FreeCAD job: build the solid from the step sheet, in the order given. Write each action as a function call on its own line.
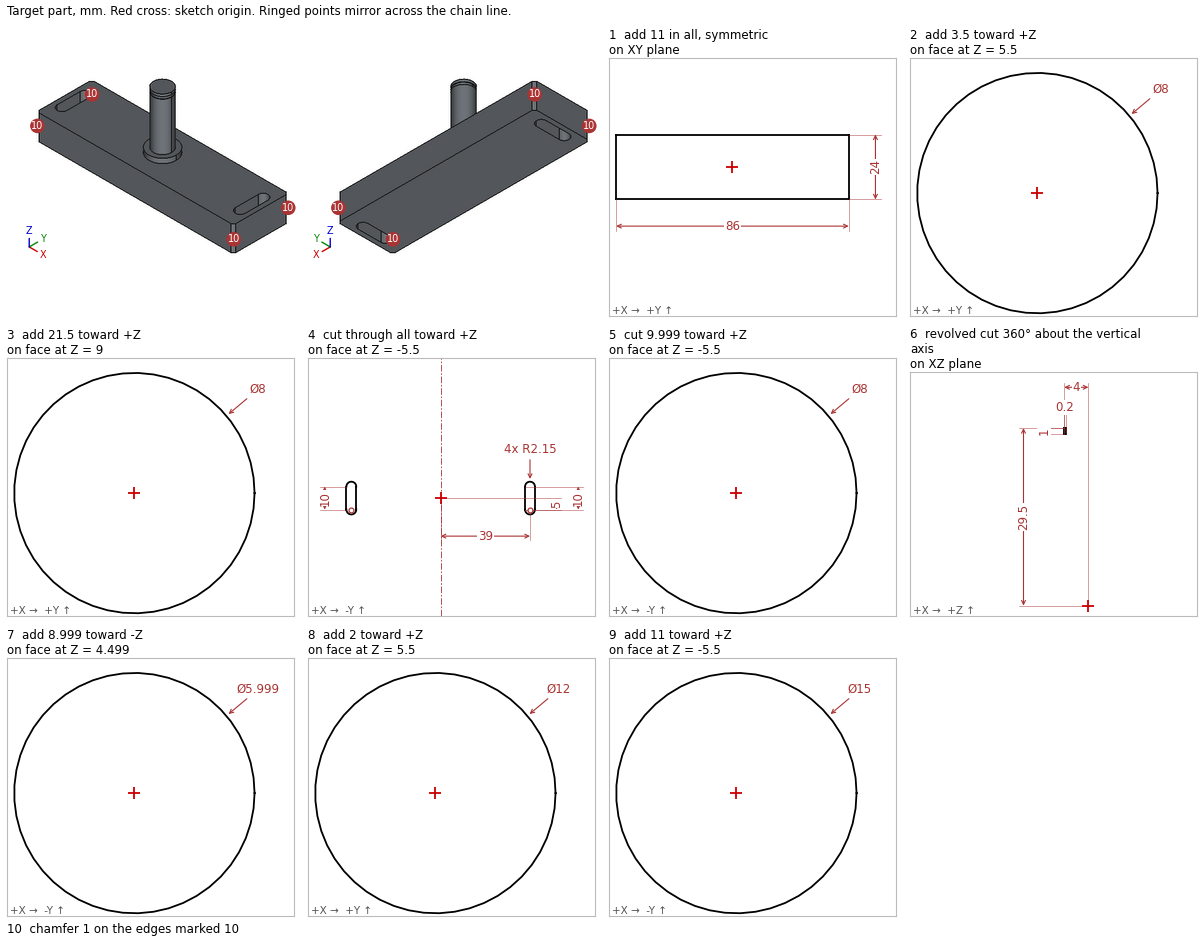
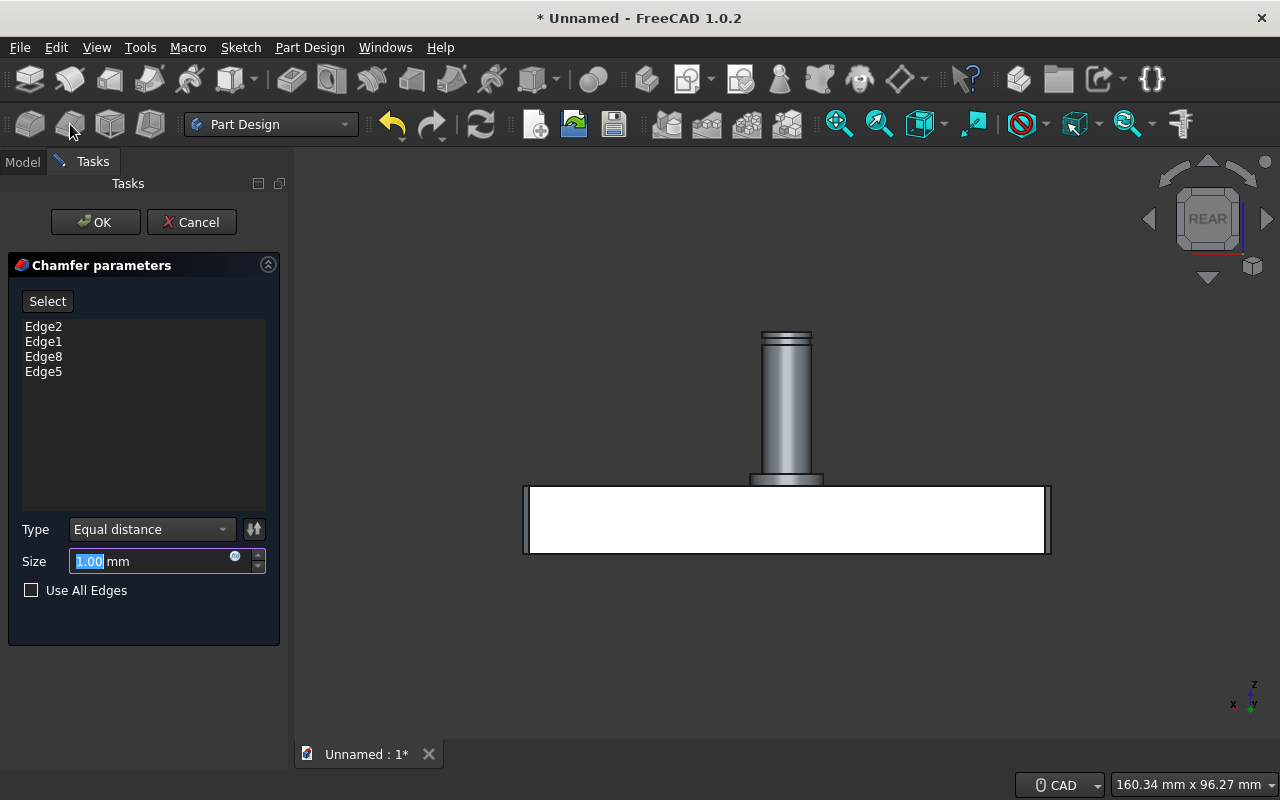
text(1)
key(Tab)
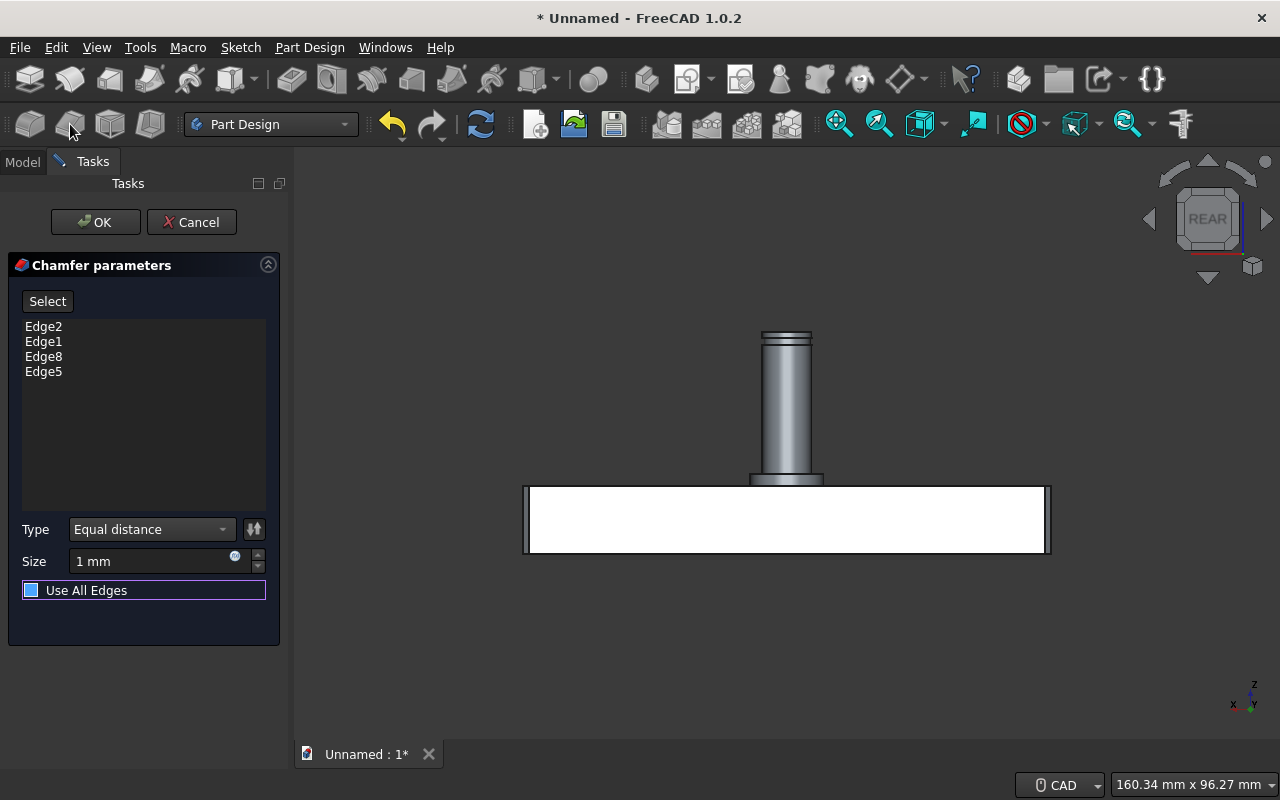
click(96, 222)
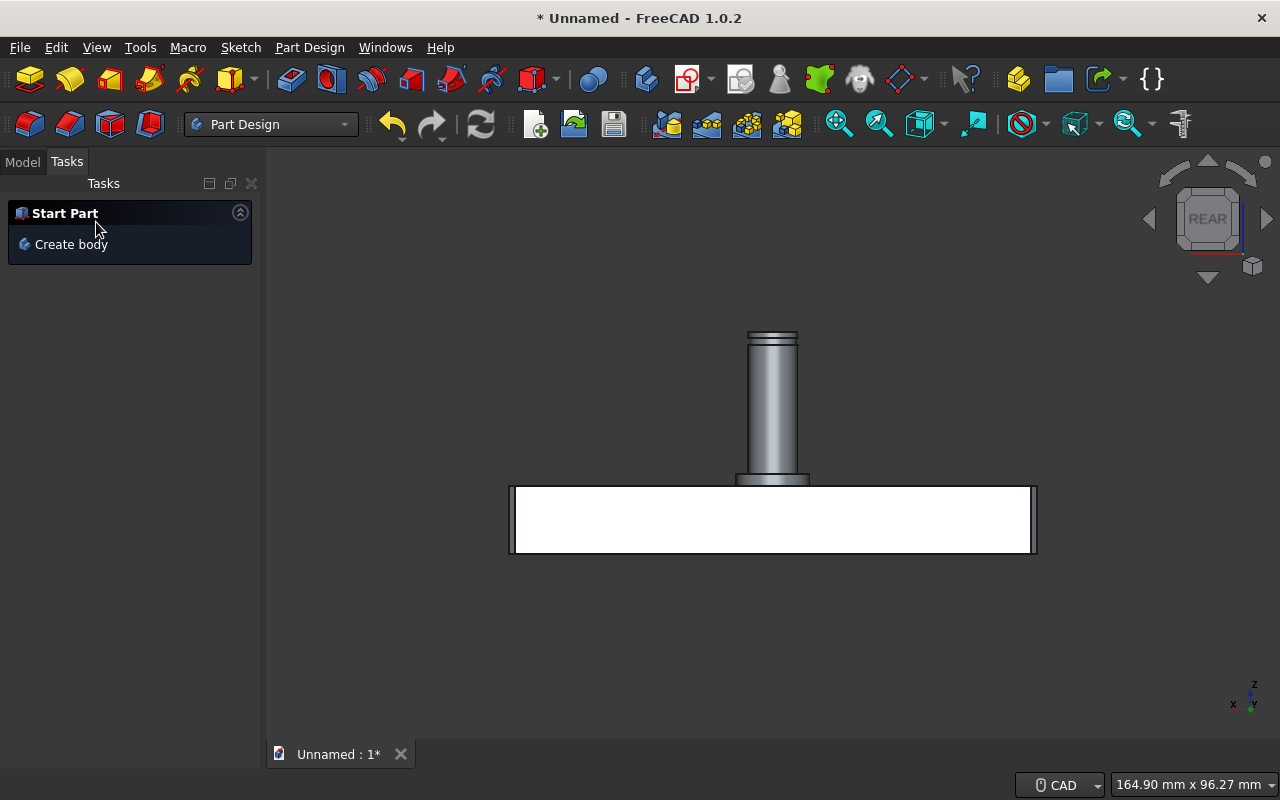
key(0)